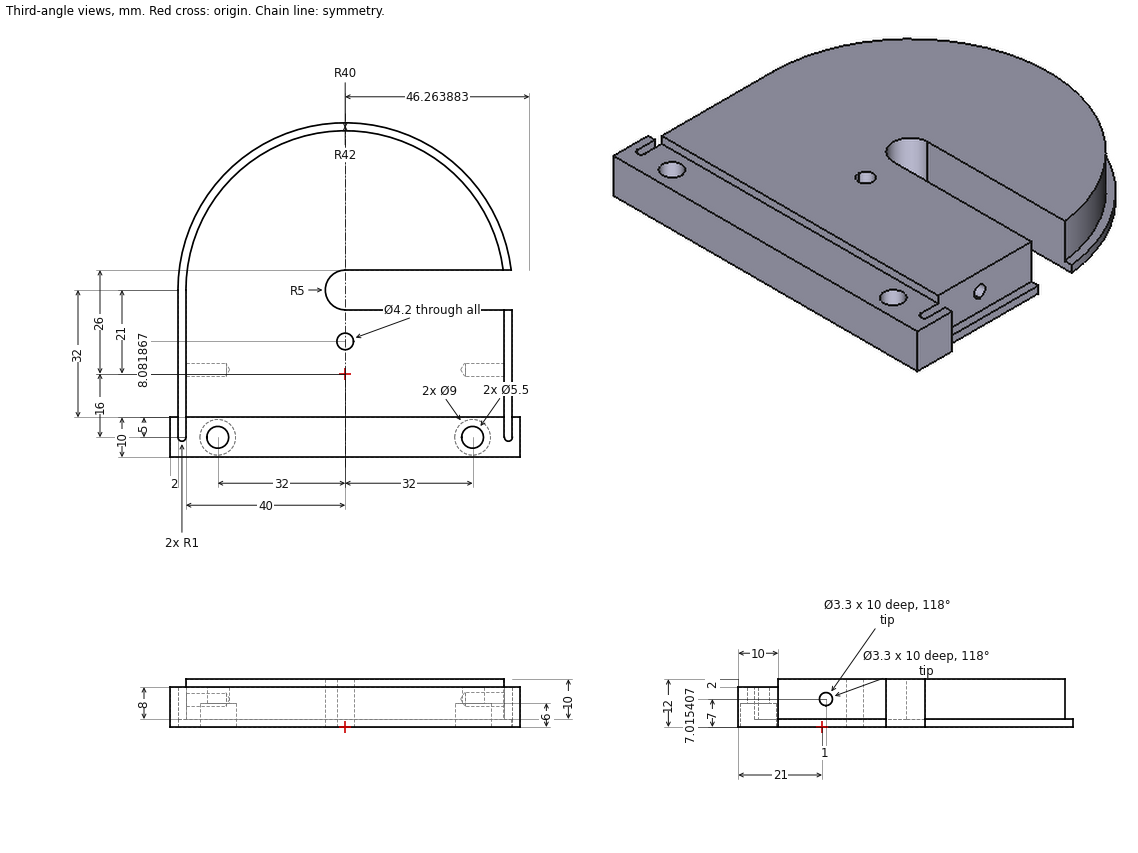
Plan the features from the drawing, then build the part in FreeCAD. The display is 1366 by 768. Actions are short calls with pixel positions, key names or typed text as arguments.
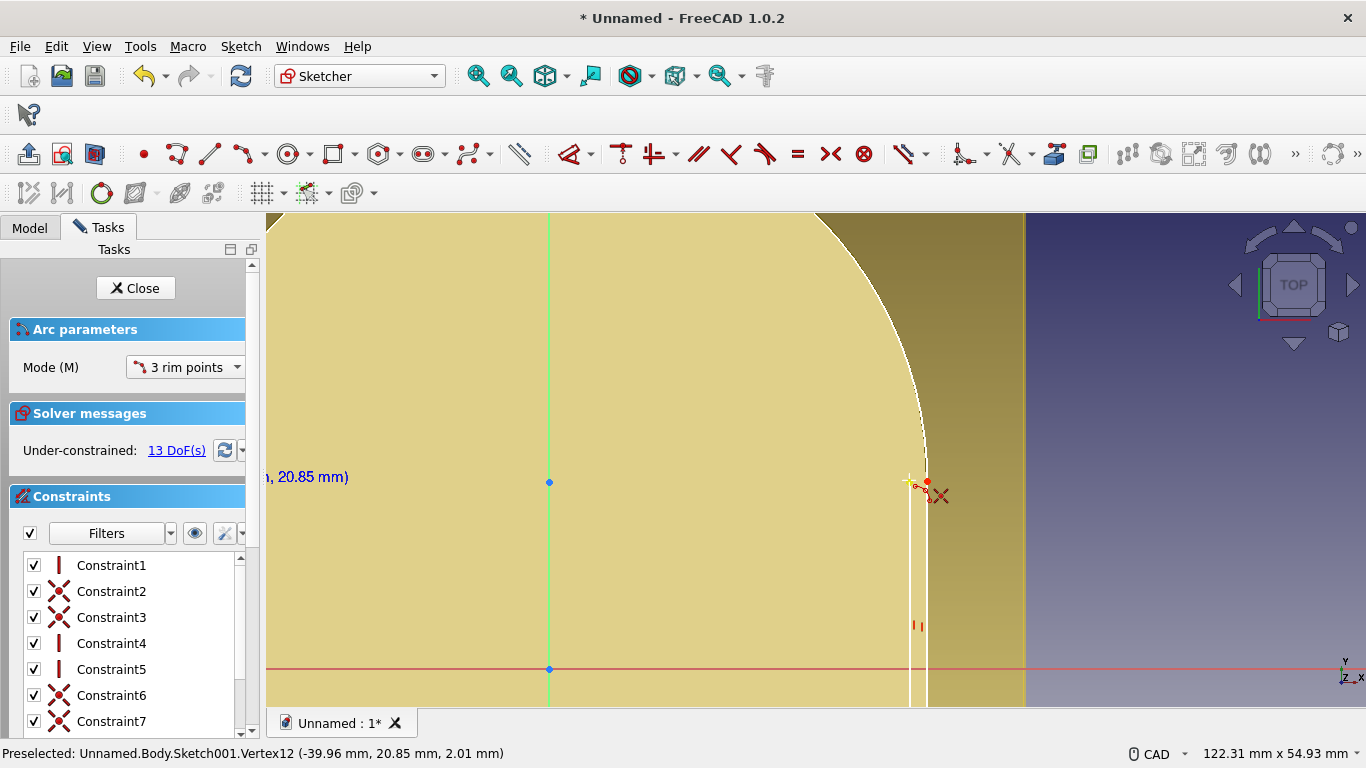
click(910, 482)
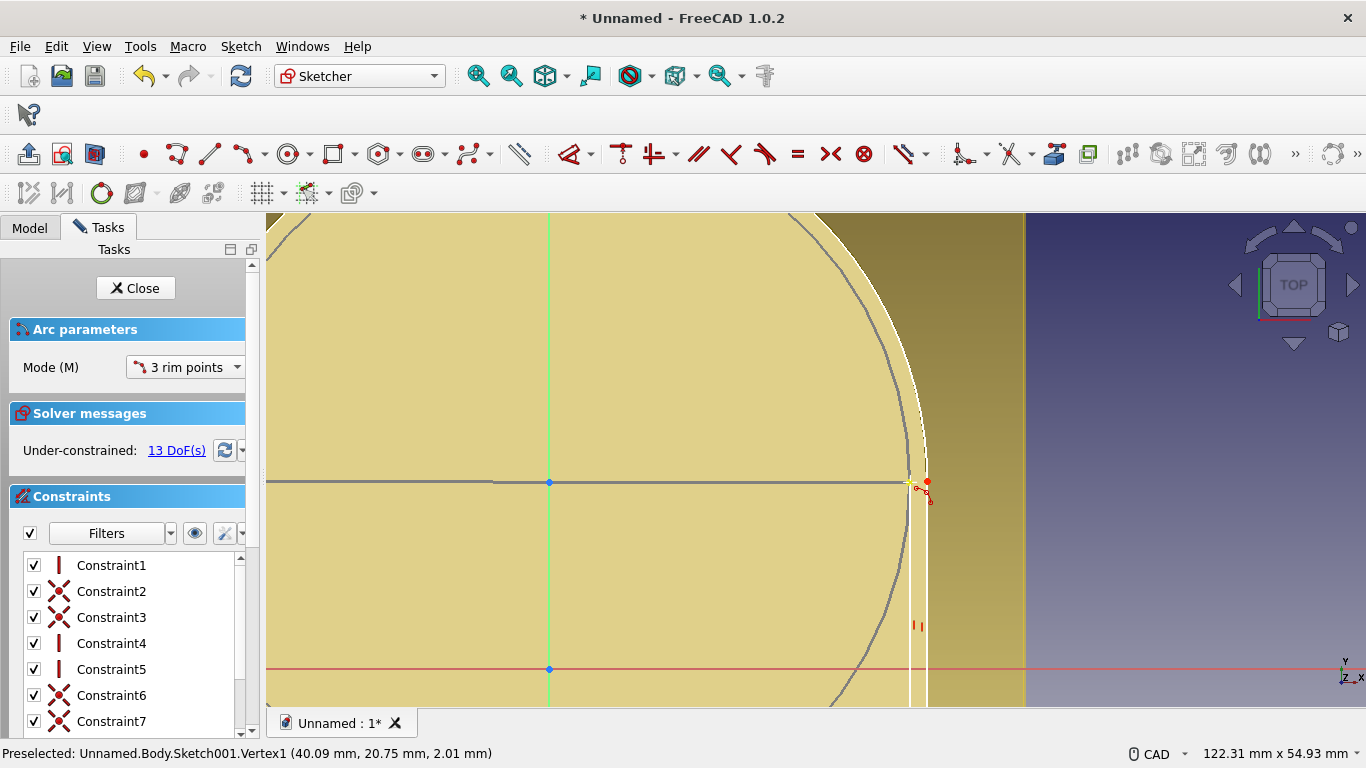
scroll(909, 480, down, 4)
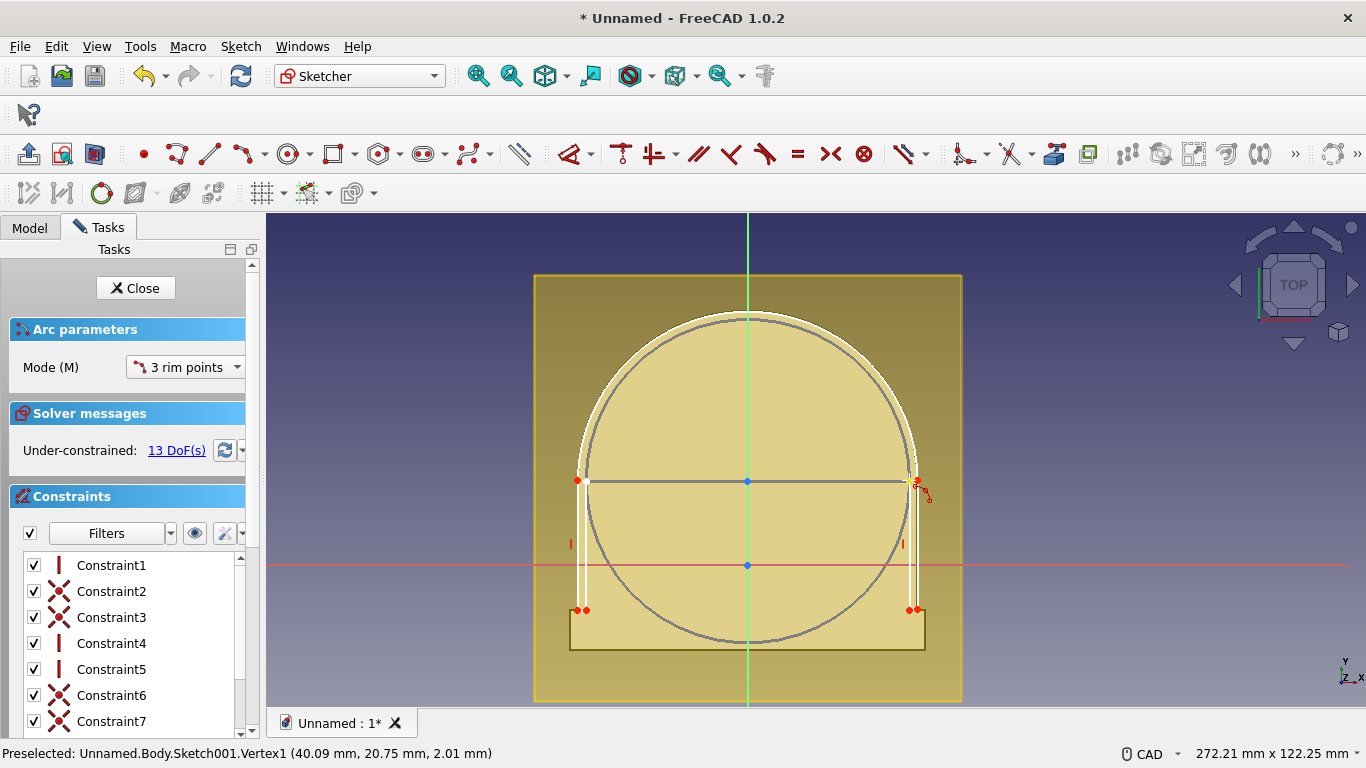
scroll(798, 327, up, 4)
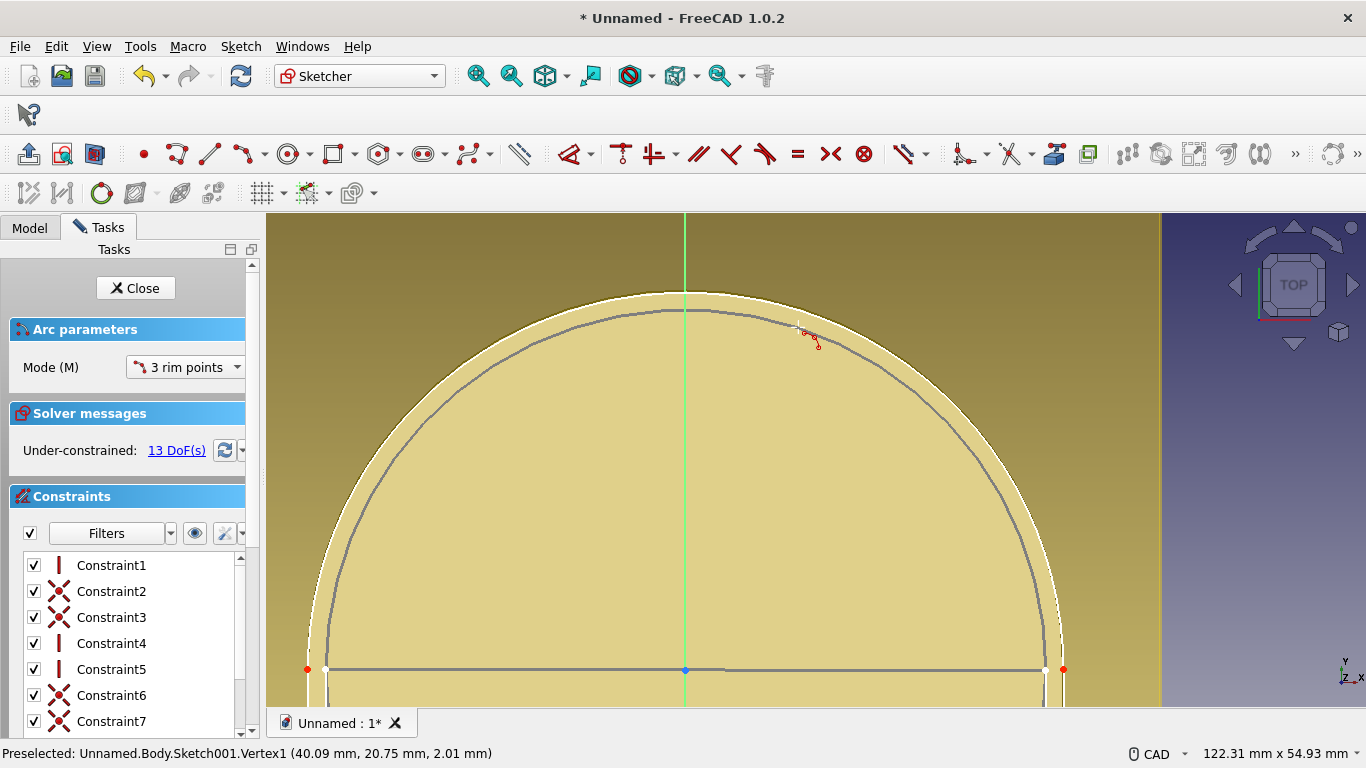
click(797, 326)
key(Escape)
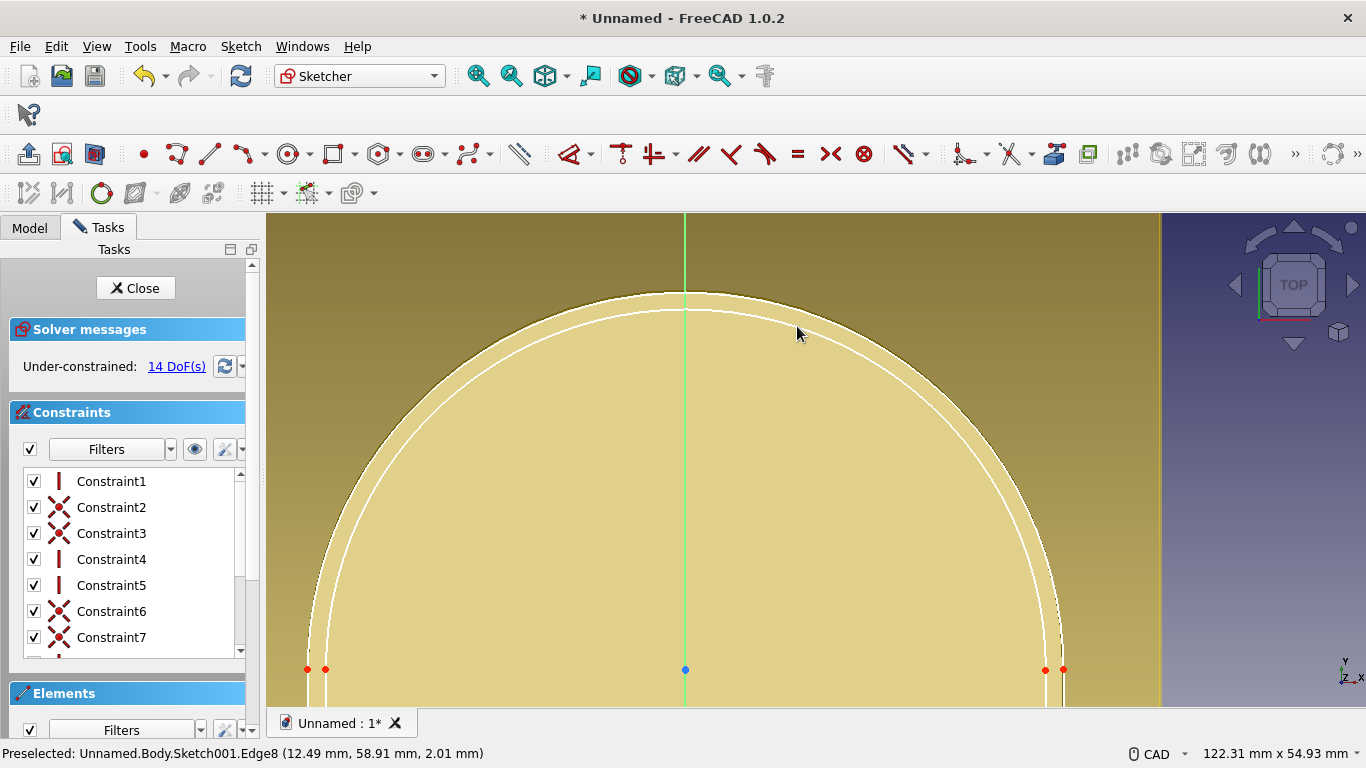
scroll(798, 327, down, 4)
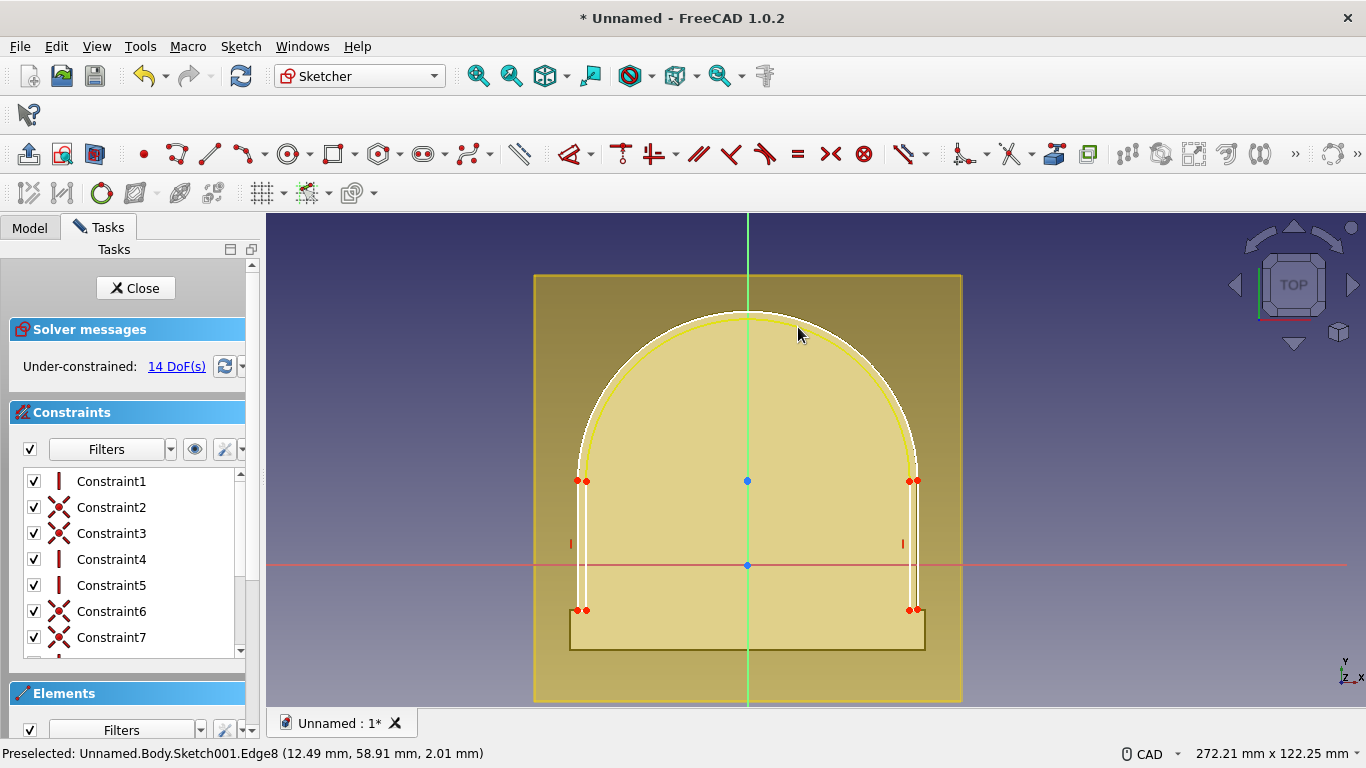
scroll(914, 610, up, 7)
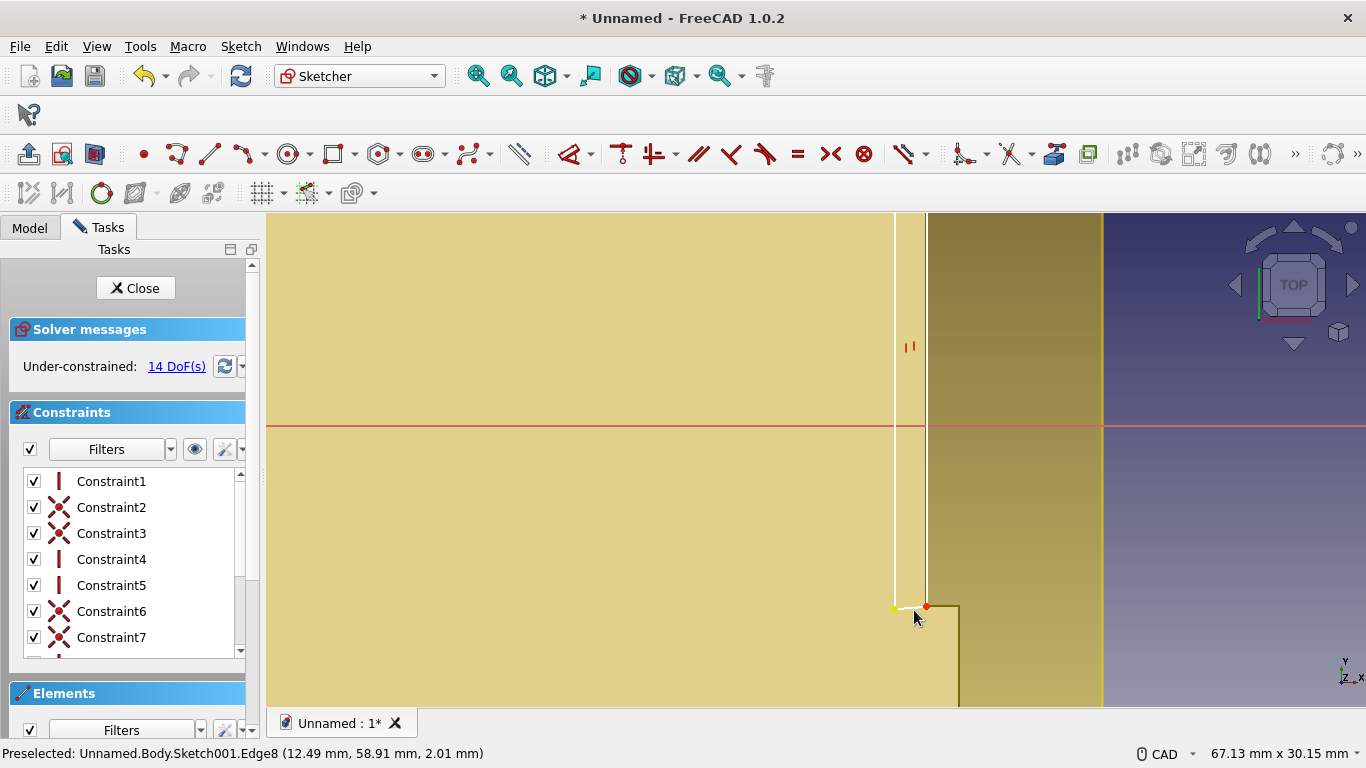
click(911, 608)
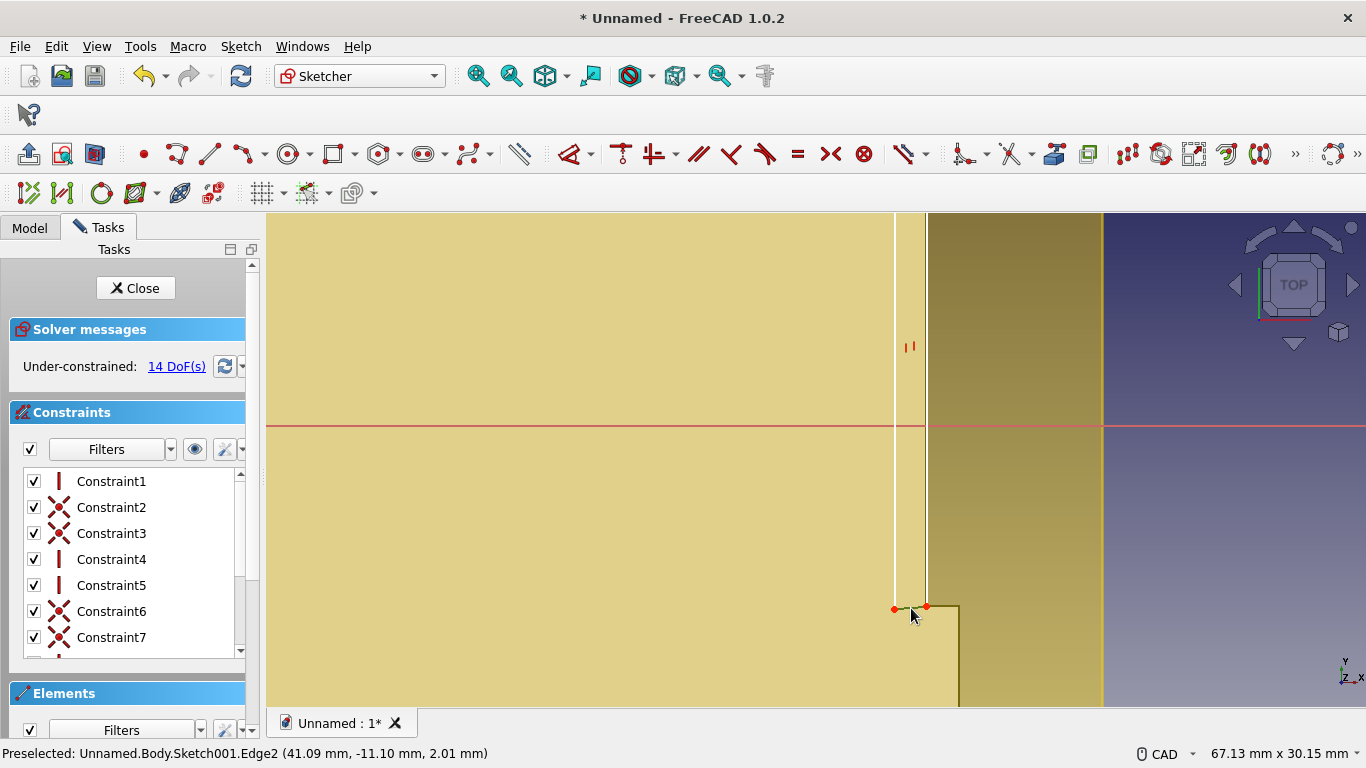
click(676, 154)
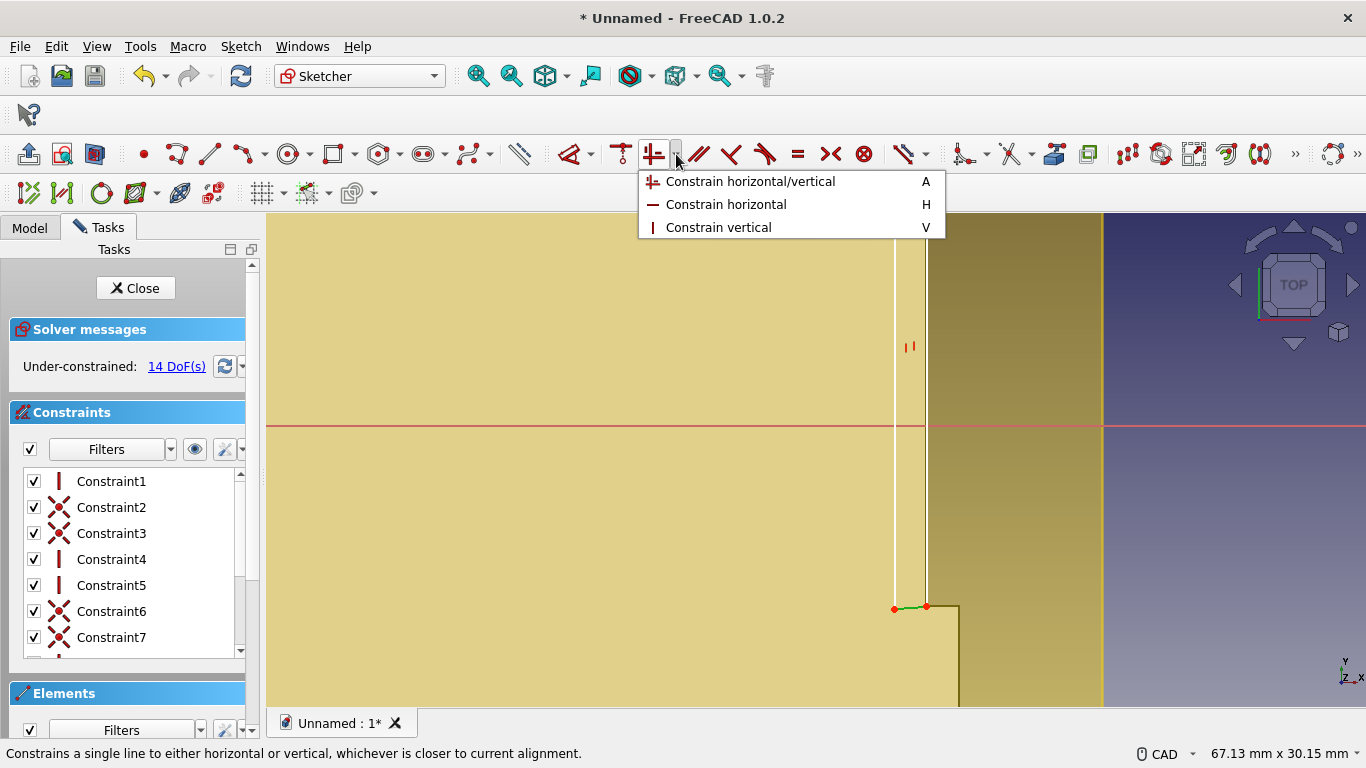
click(792, 204)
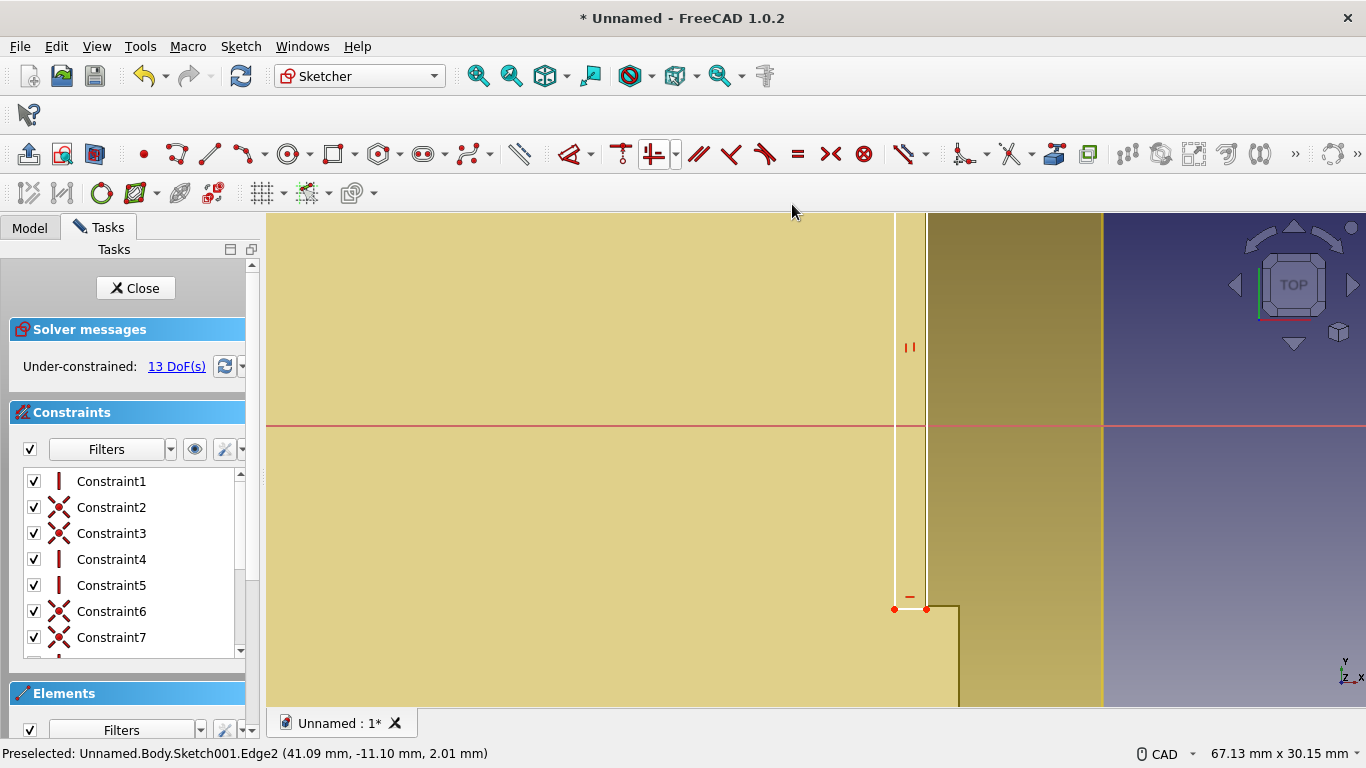
scroll(914, 611, down, 7)